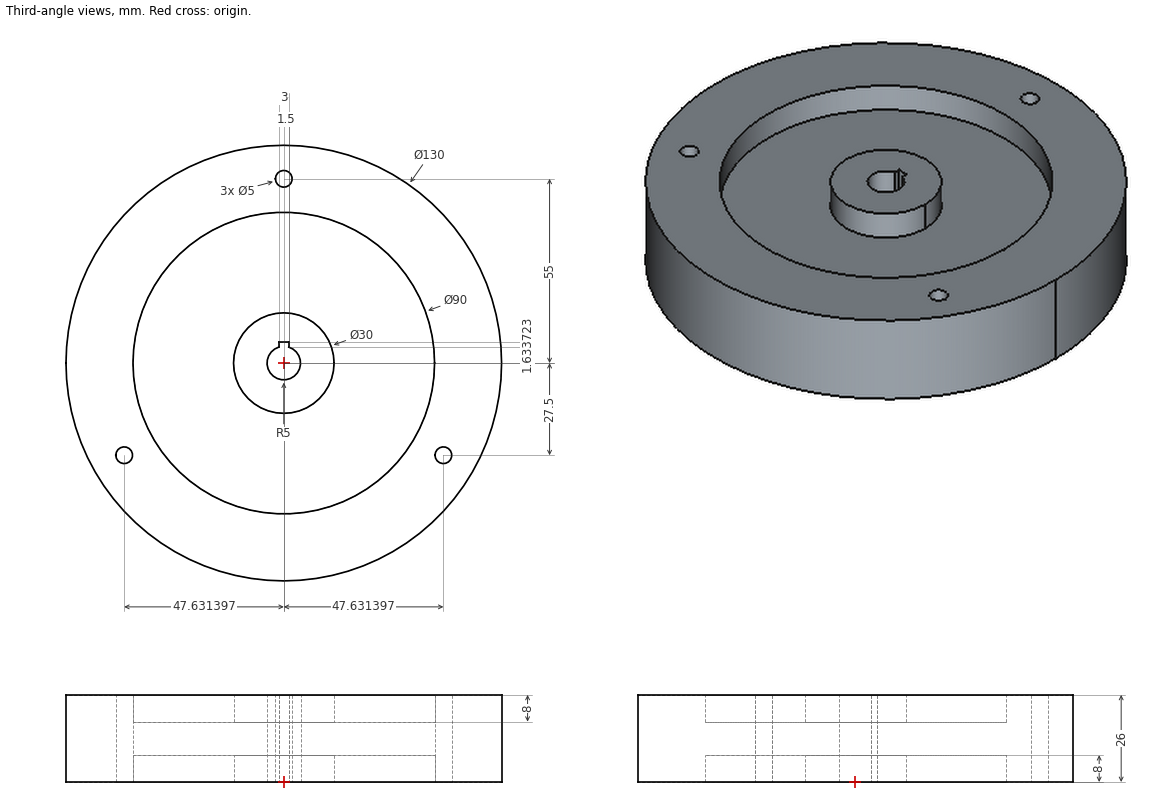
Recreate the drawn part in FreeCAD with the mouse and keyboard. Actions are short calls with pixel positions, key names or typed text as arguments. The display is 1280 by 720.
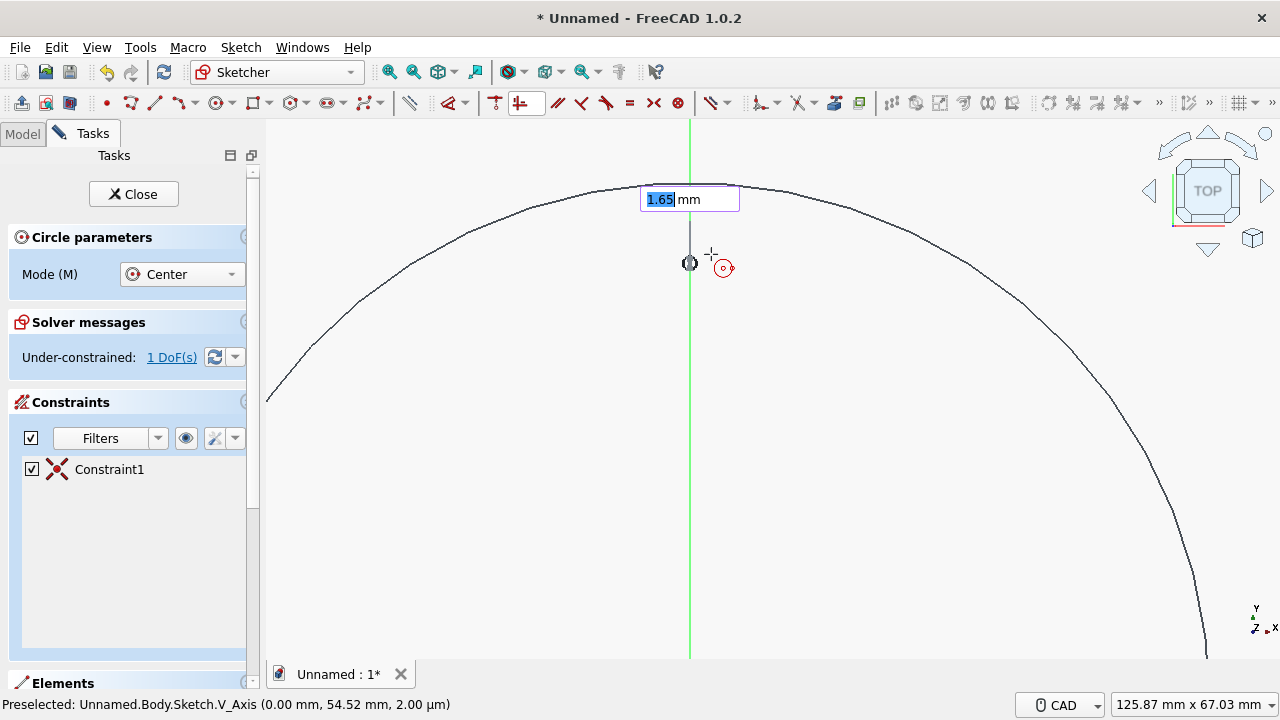
click(709, 253)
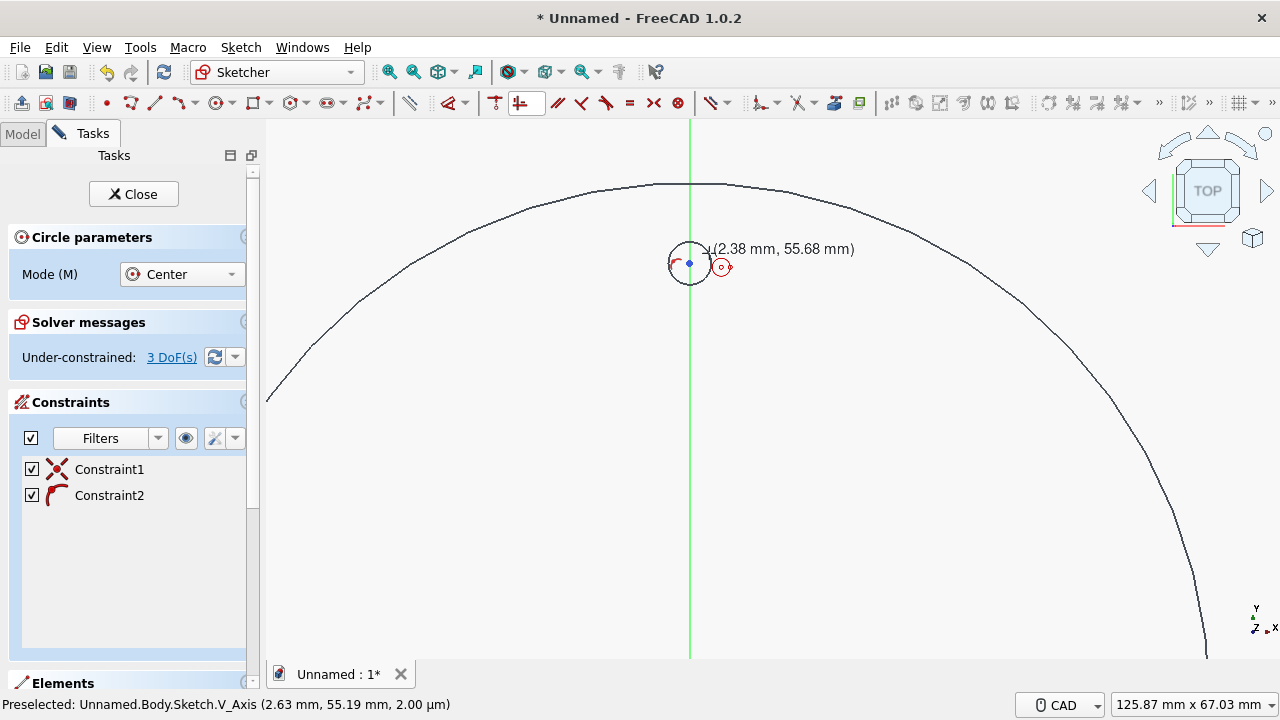
scroll(711, 254, down, 6)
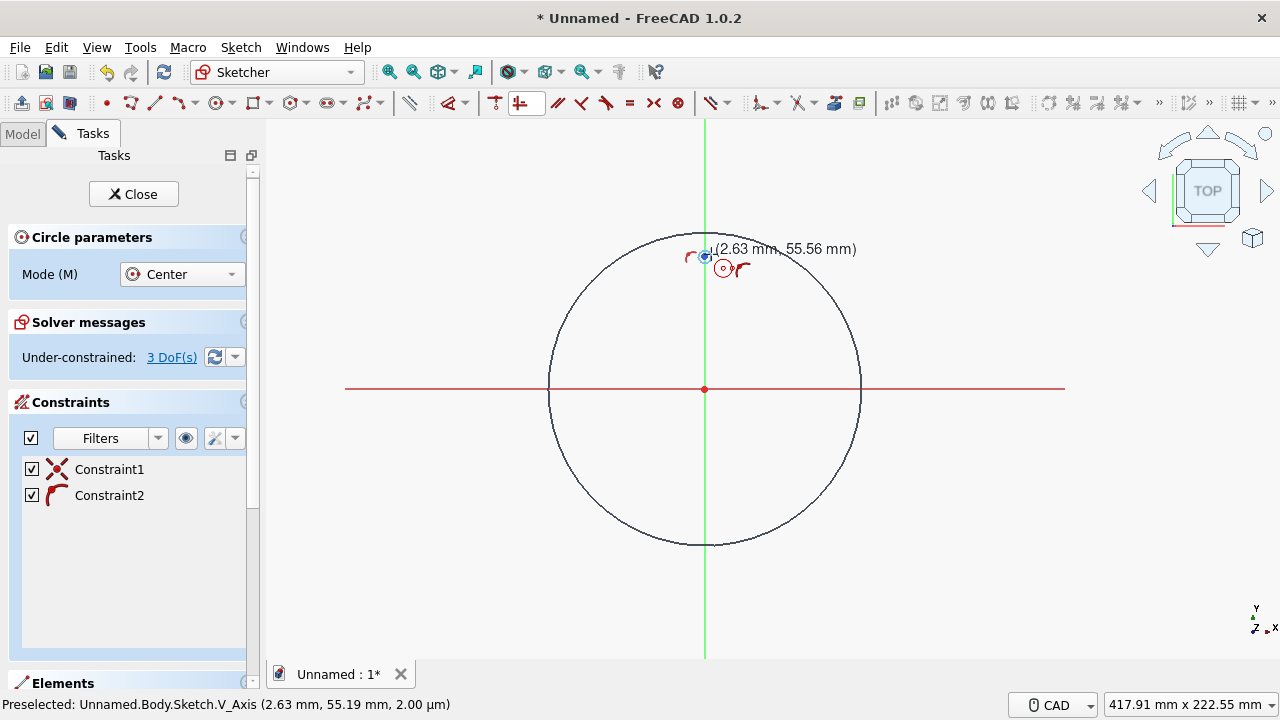
scroll(820, 456, up, 7)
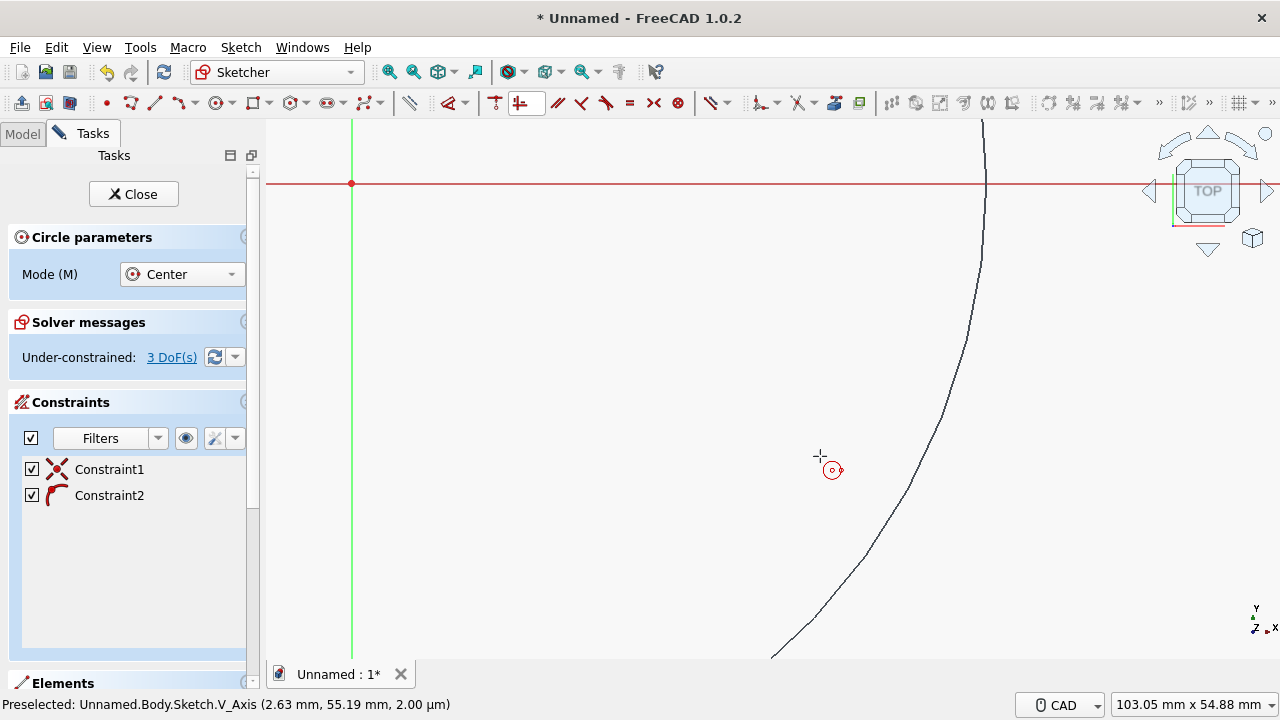
scroll(820, 456, down, 7)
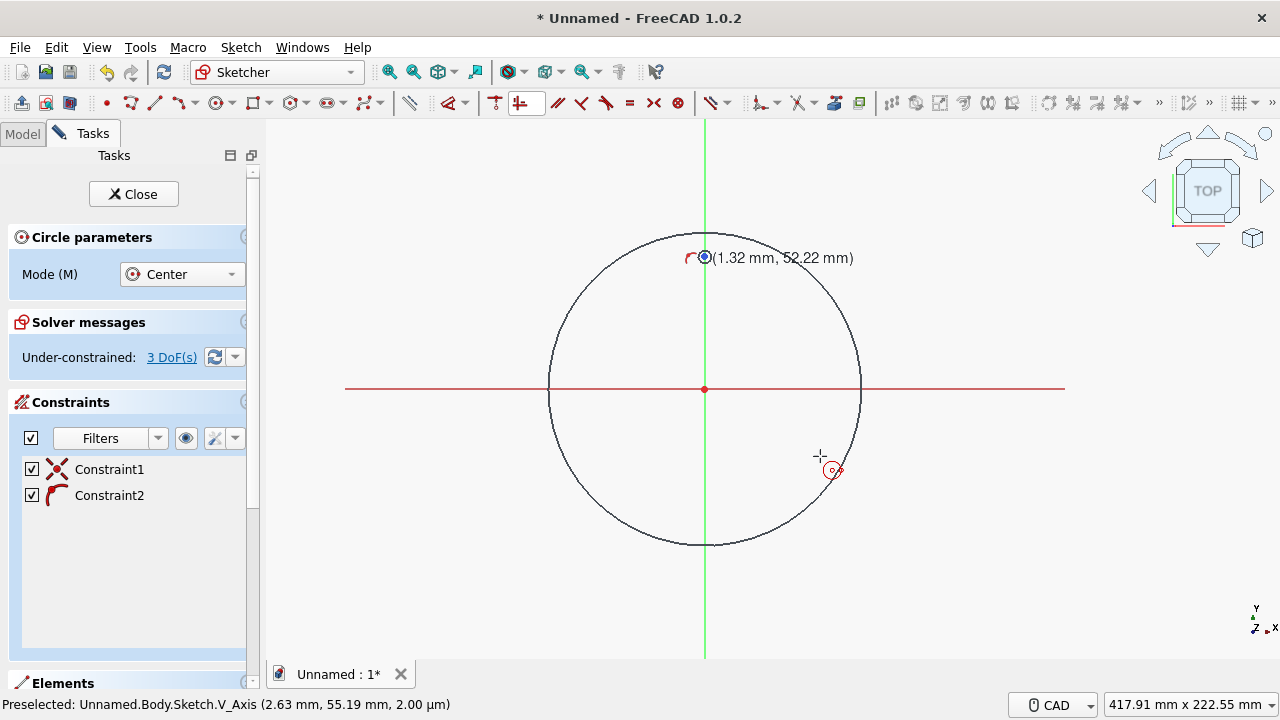
click(820, 456)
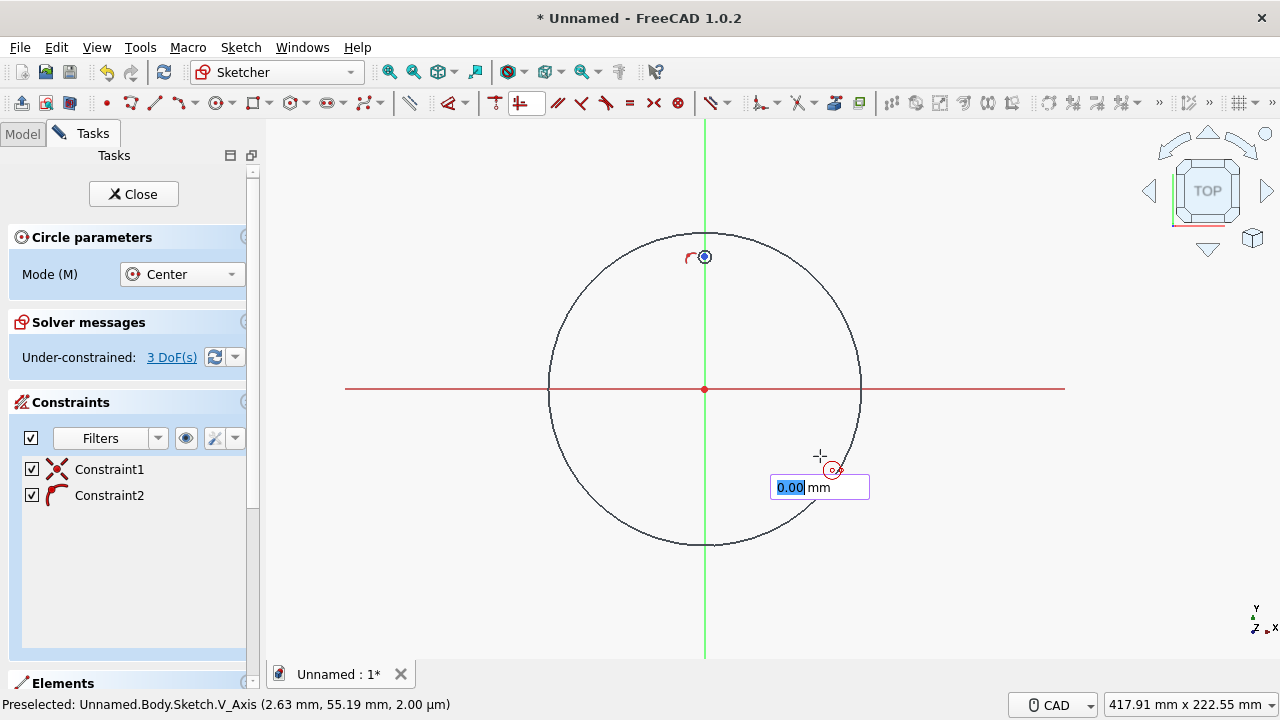
scroll(825, 452, up, 5)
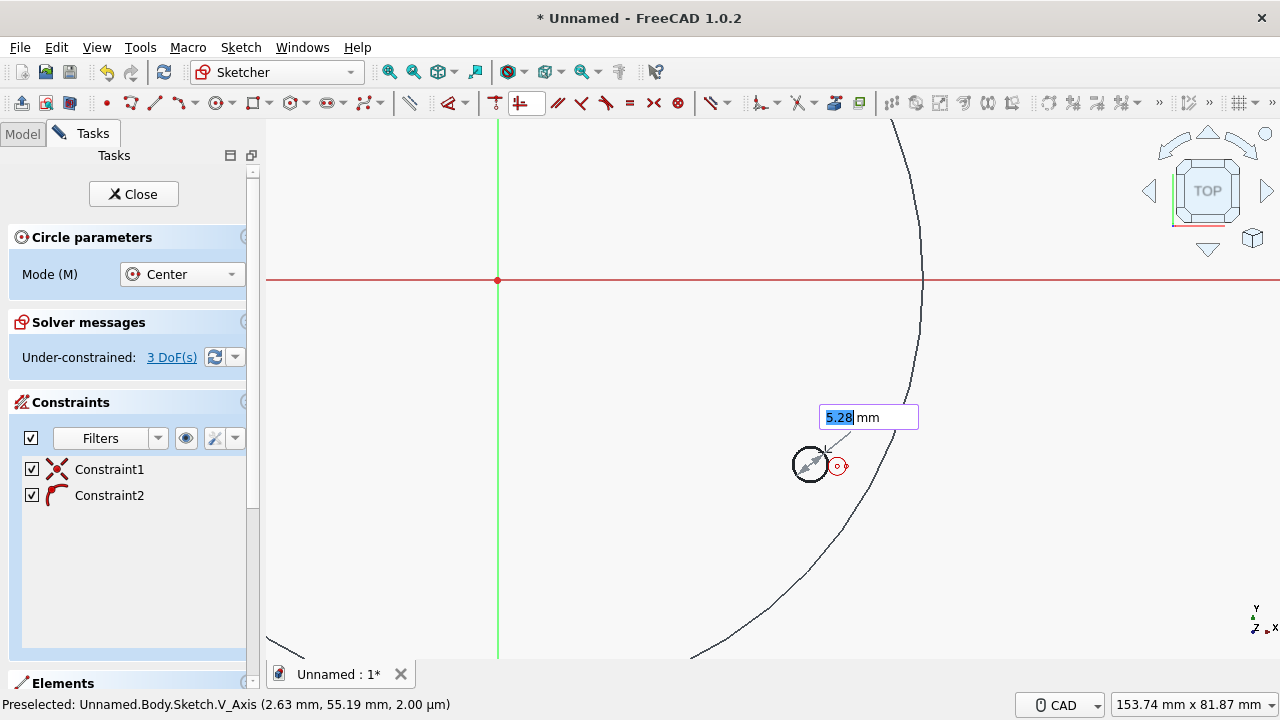
click(823, 450)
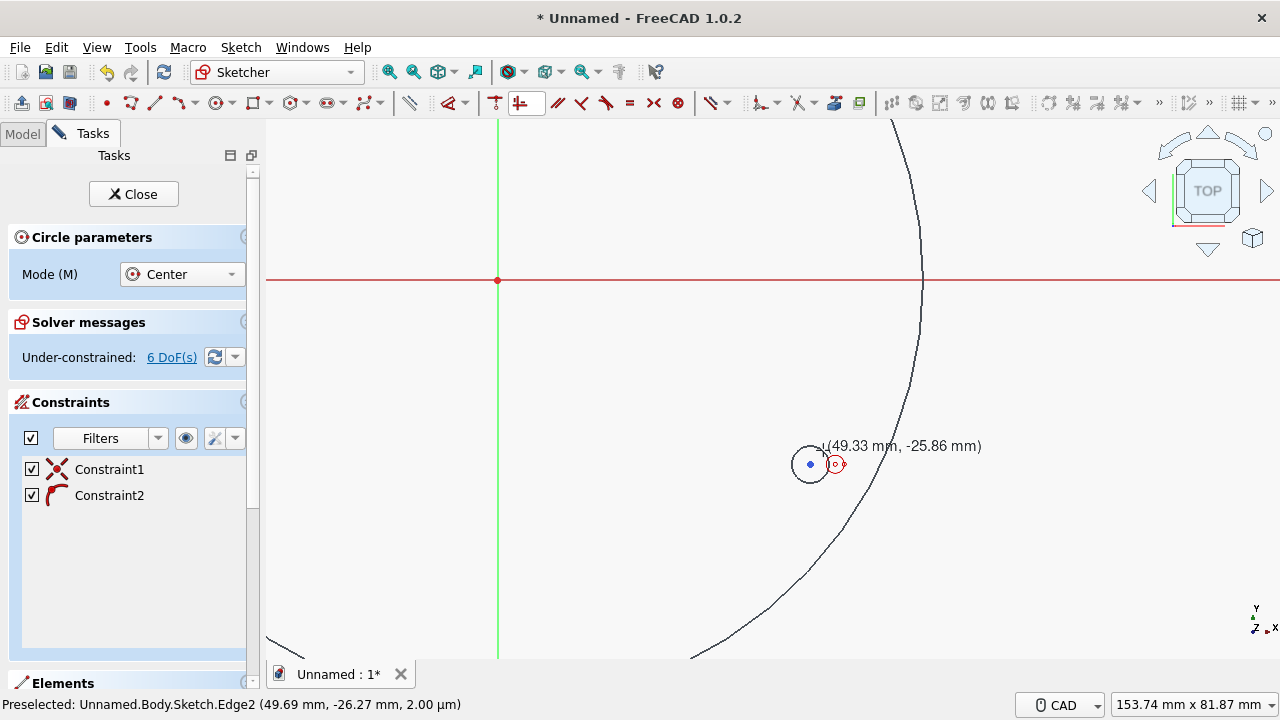
scroll(825, 452, down, 5)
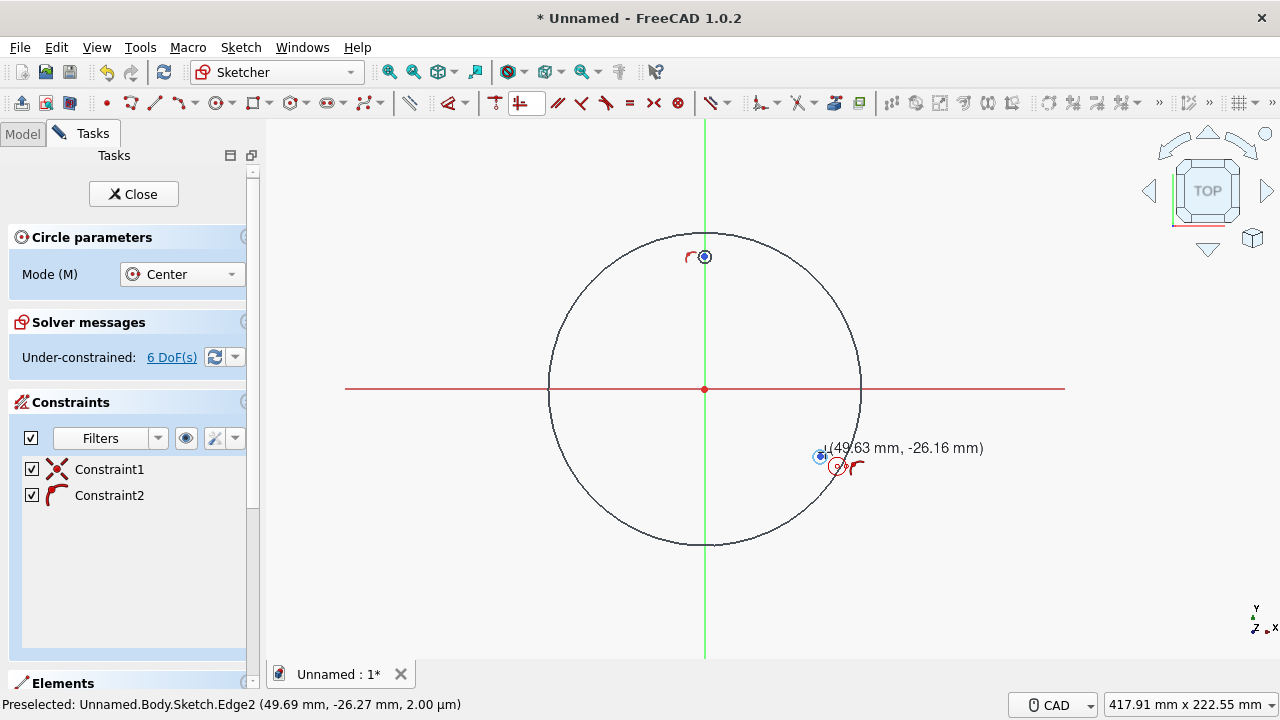
scroll(589, 456, up, 7)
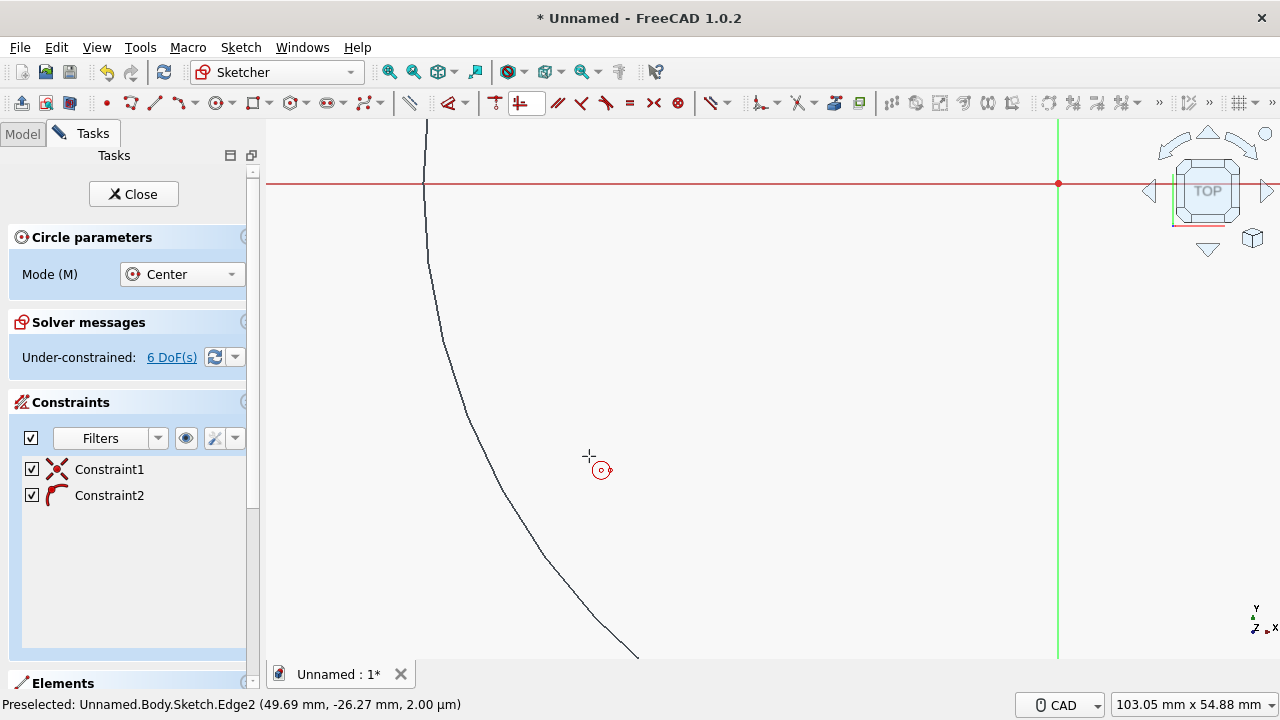
scroll(589, 456, down, 7)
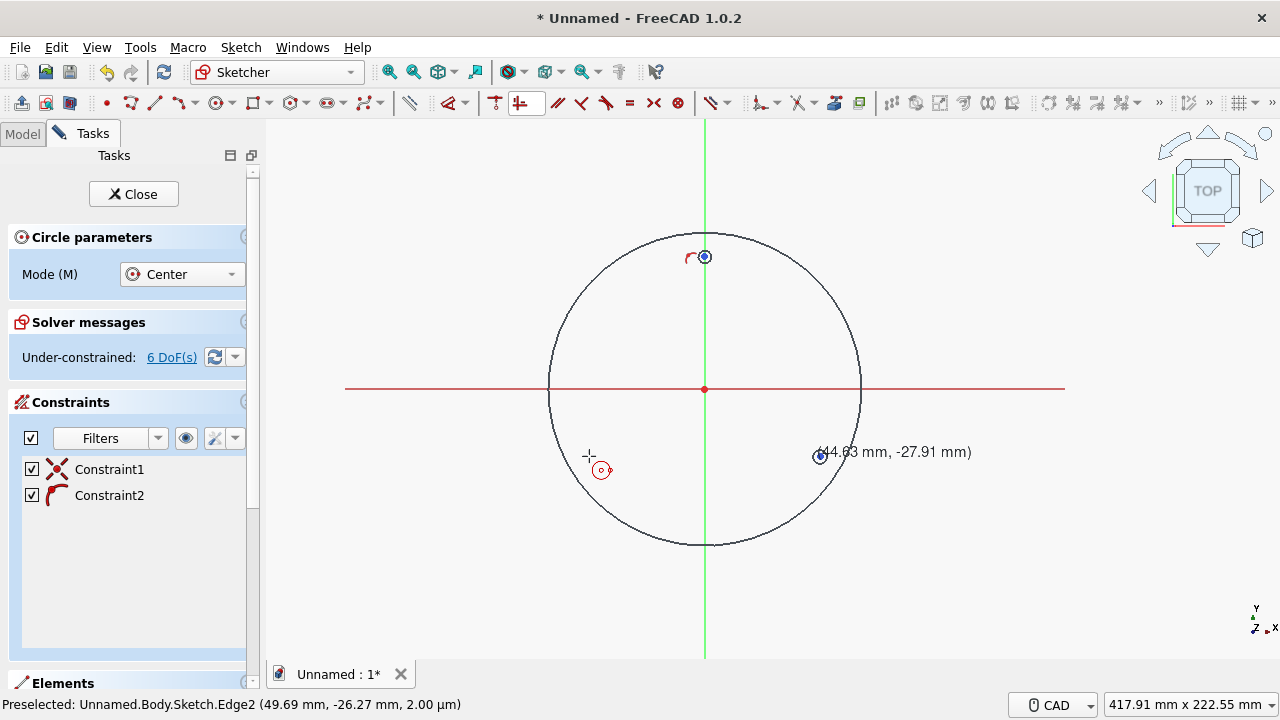
click(589, 456)